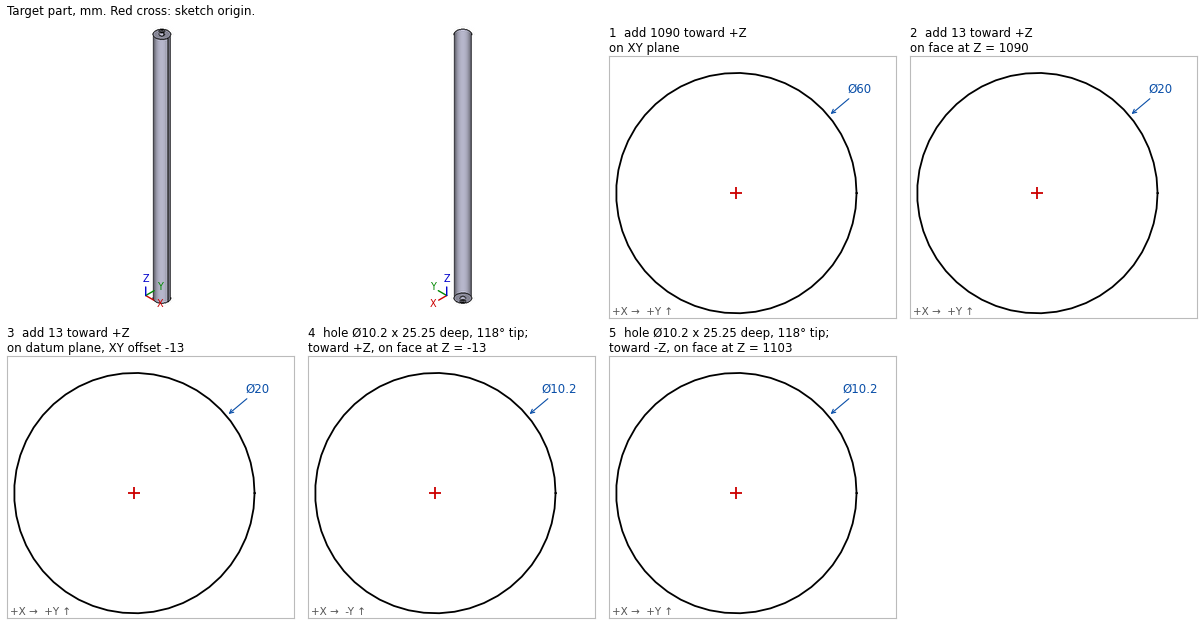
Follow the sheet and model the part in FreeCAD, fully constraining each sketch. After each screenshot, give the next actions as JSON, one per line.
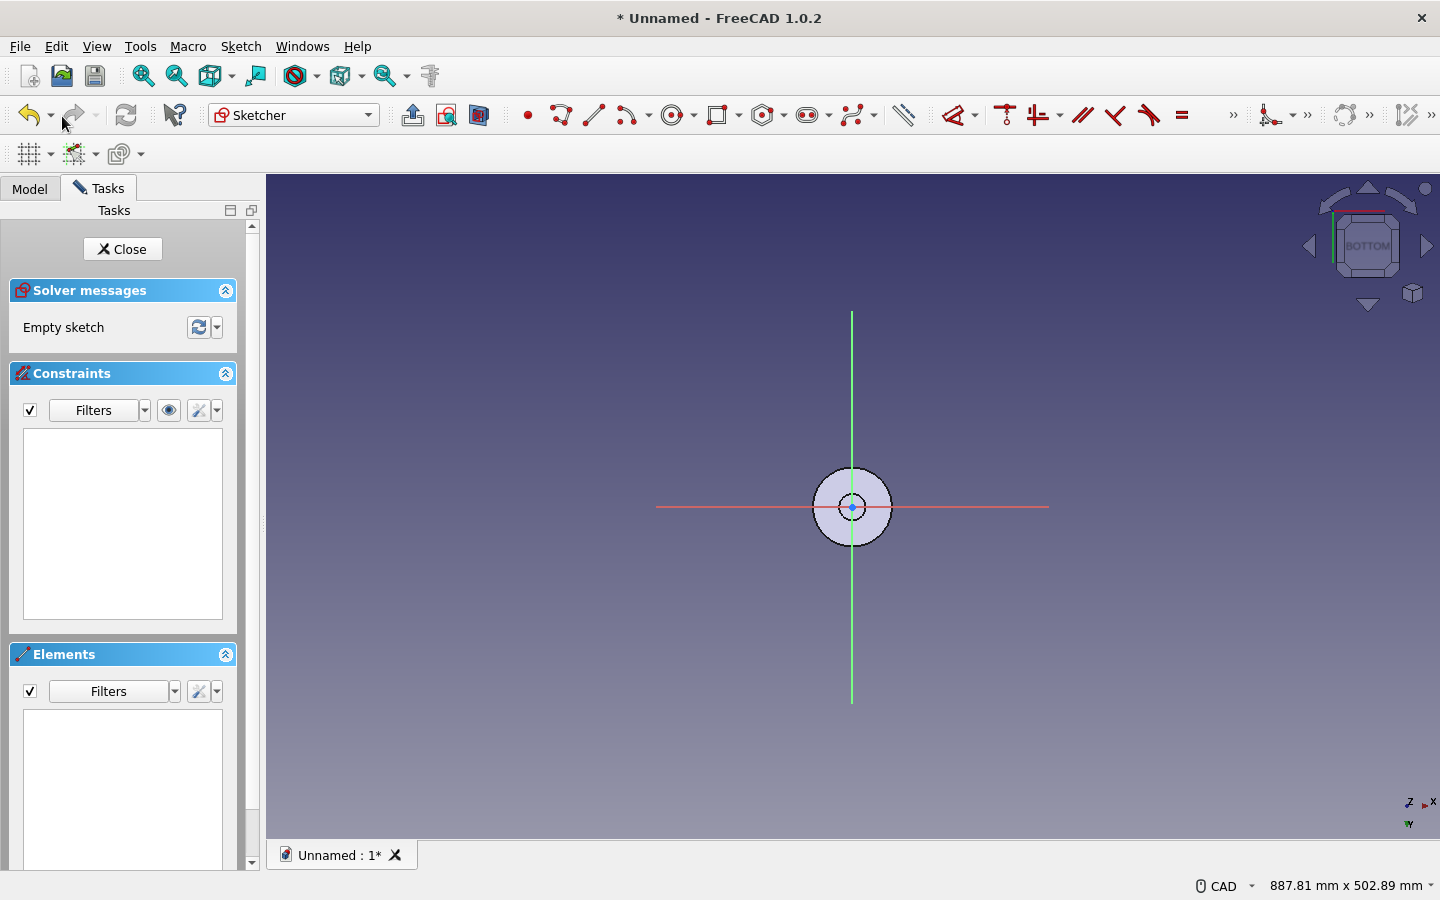
{"action": "scroll", "coordinate": [856, 507], "scroll_direction": "up", "scroll_amount": 15}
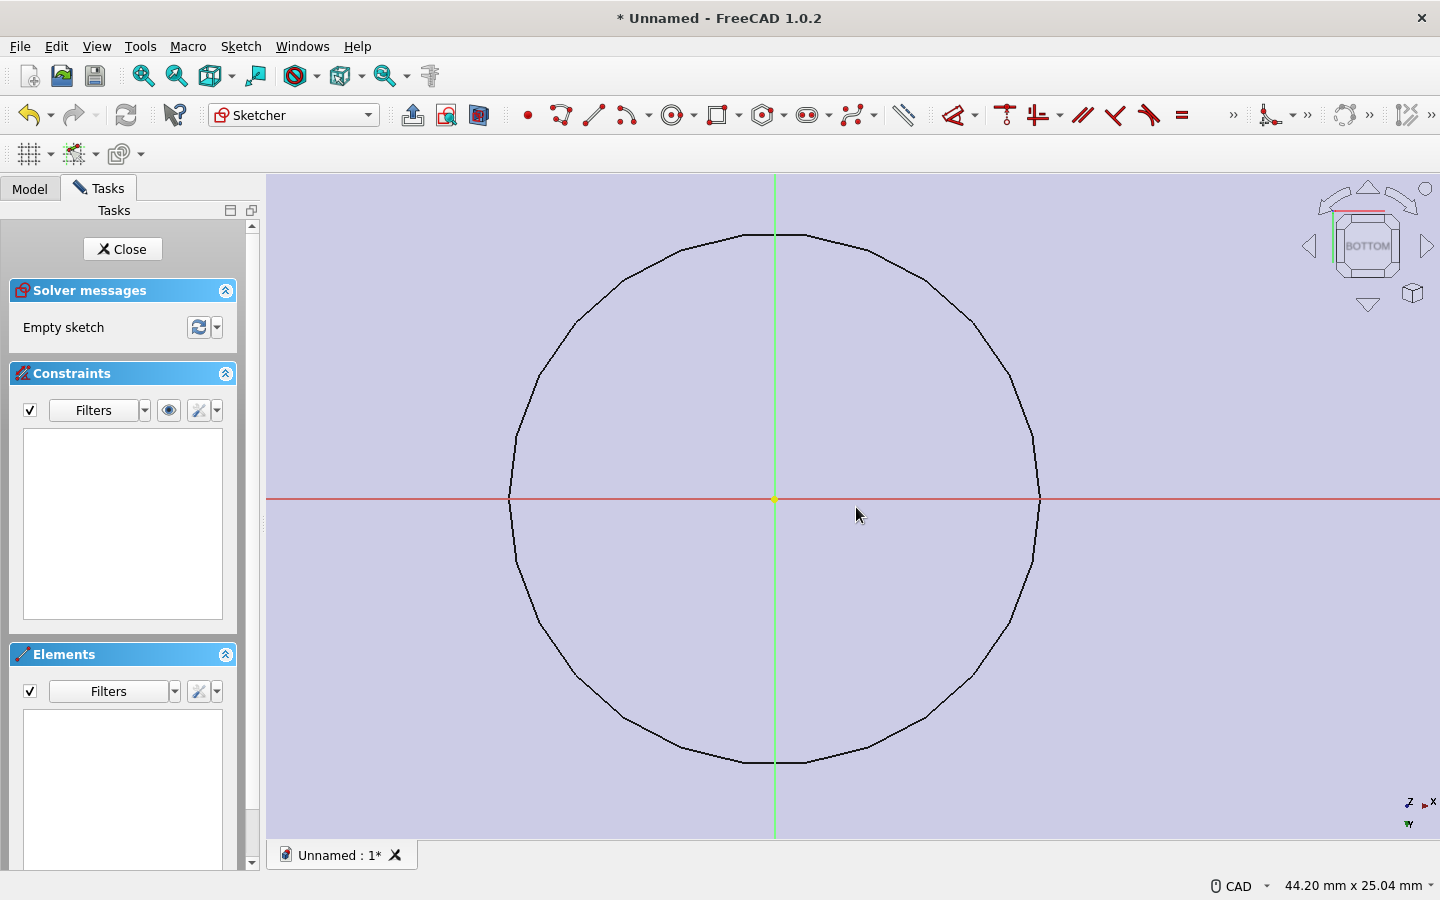
{"action": "scroll", "coordinate": [754, 484], "scroll_direction": "up", "scroll_amount": 2}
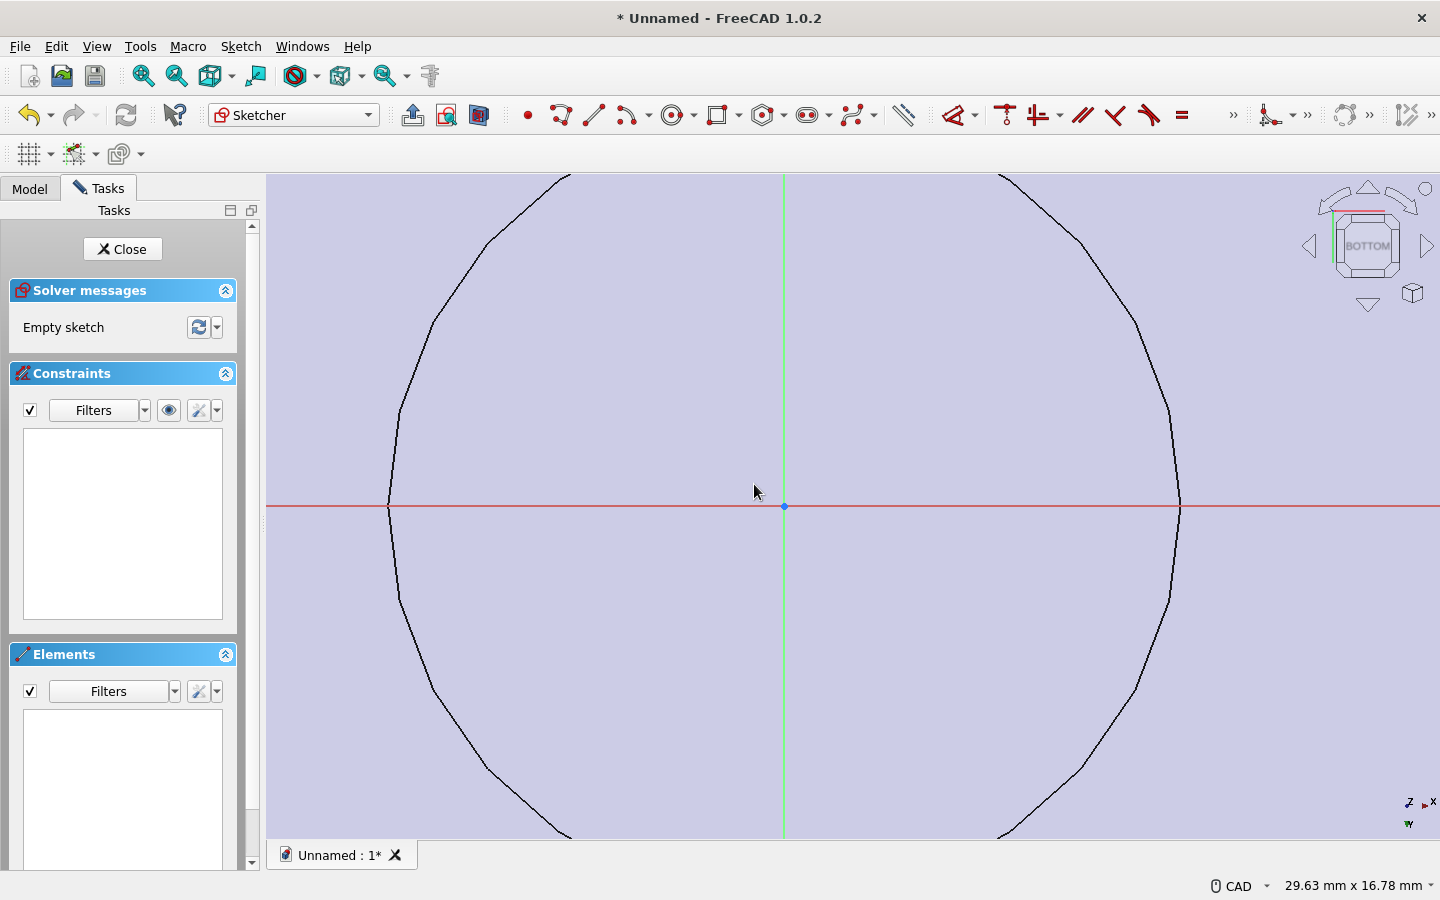
{"action": "key", "text": "g c"}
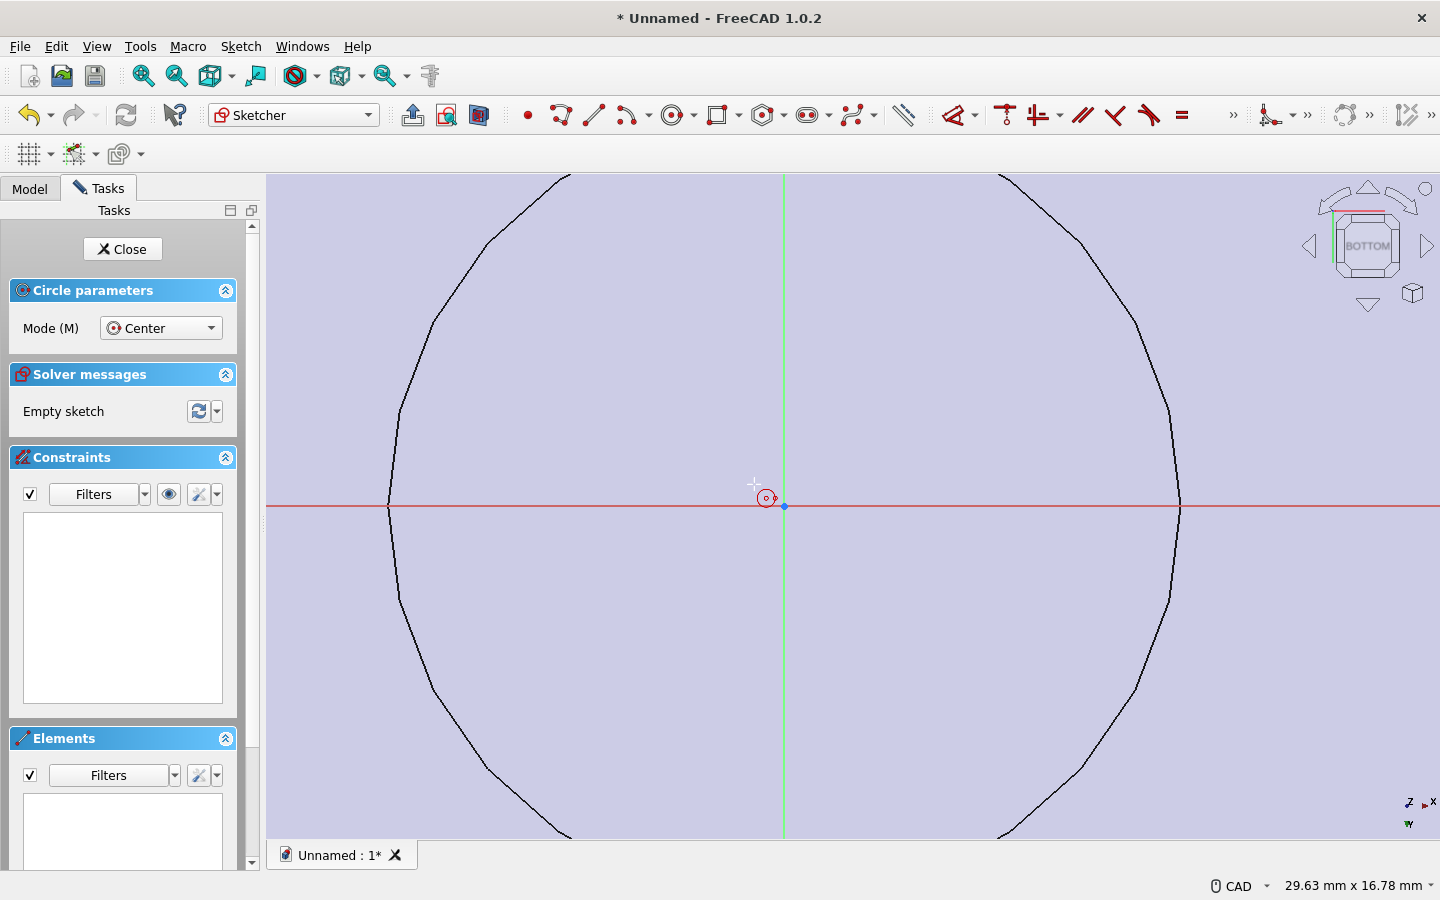
{"action": "left_click", "coordinate": [784, 506]}
{"action": "mouse_move", "coordinate": [927, 363]}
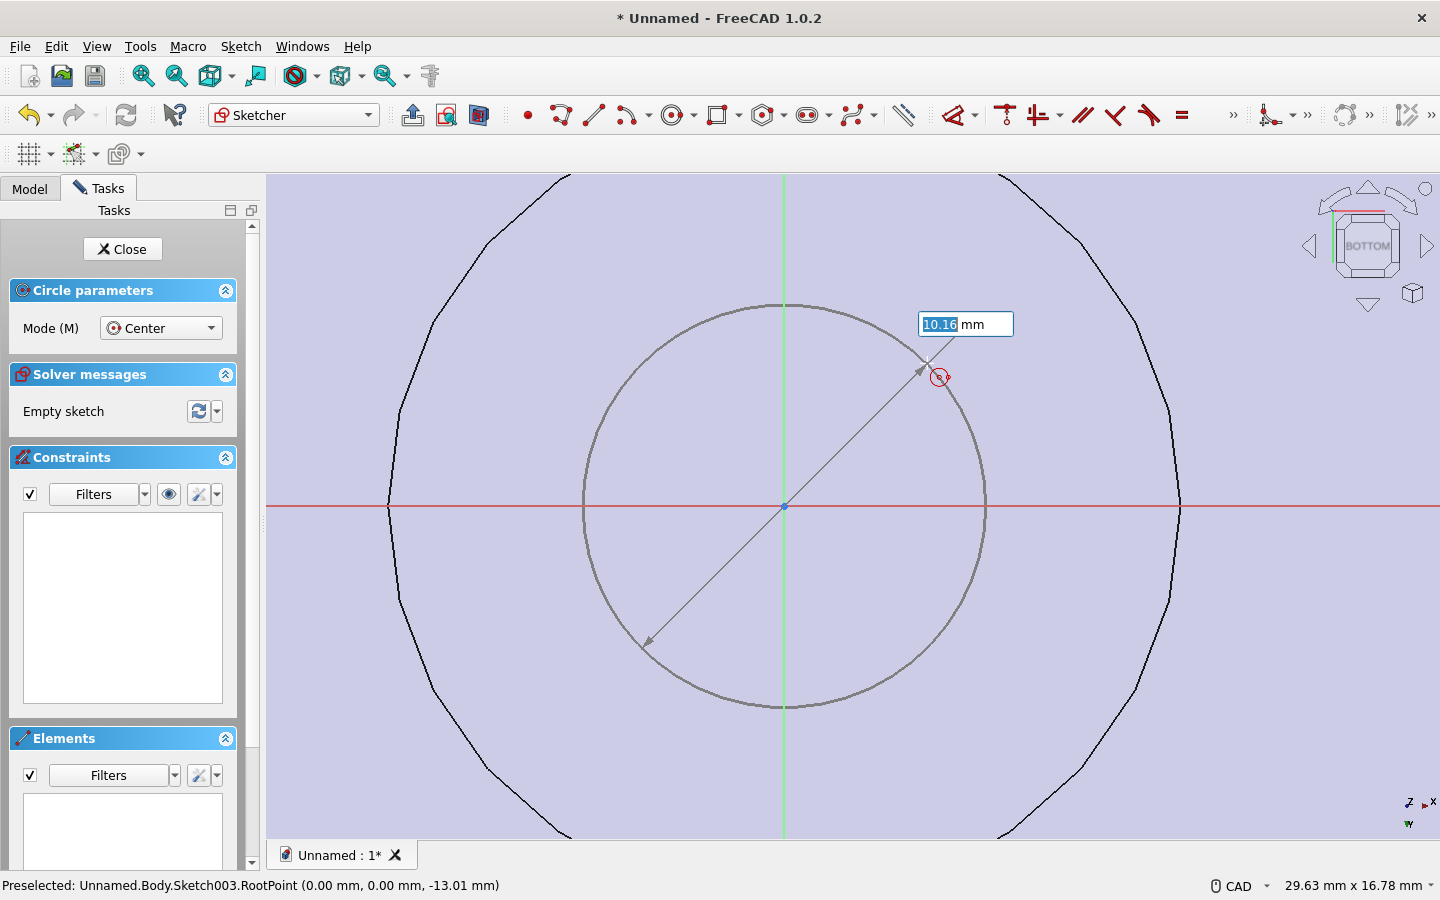
{"action": "type", "text": "10.2"}
{"action": "key", "text": "Return"}
{"action": "key", "text": "Escape"}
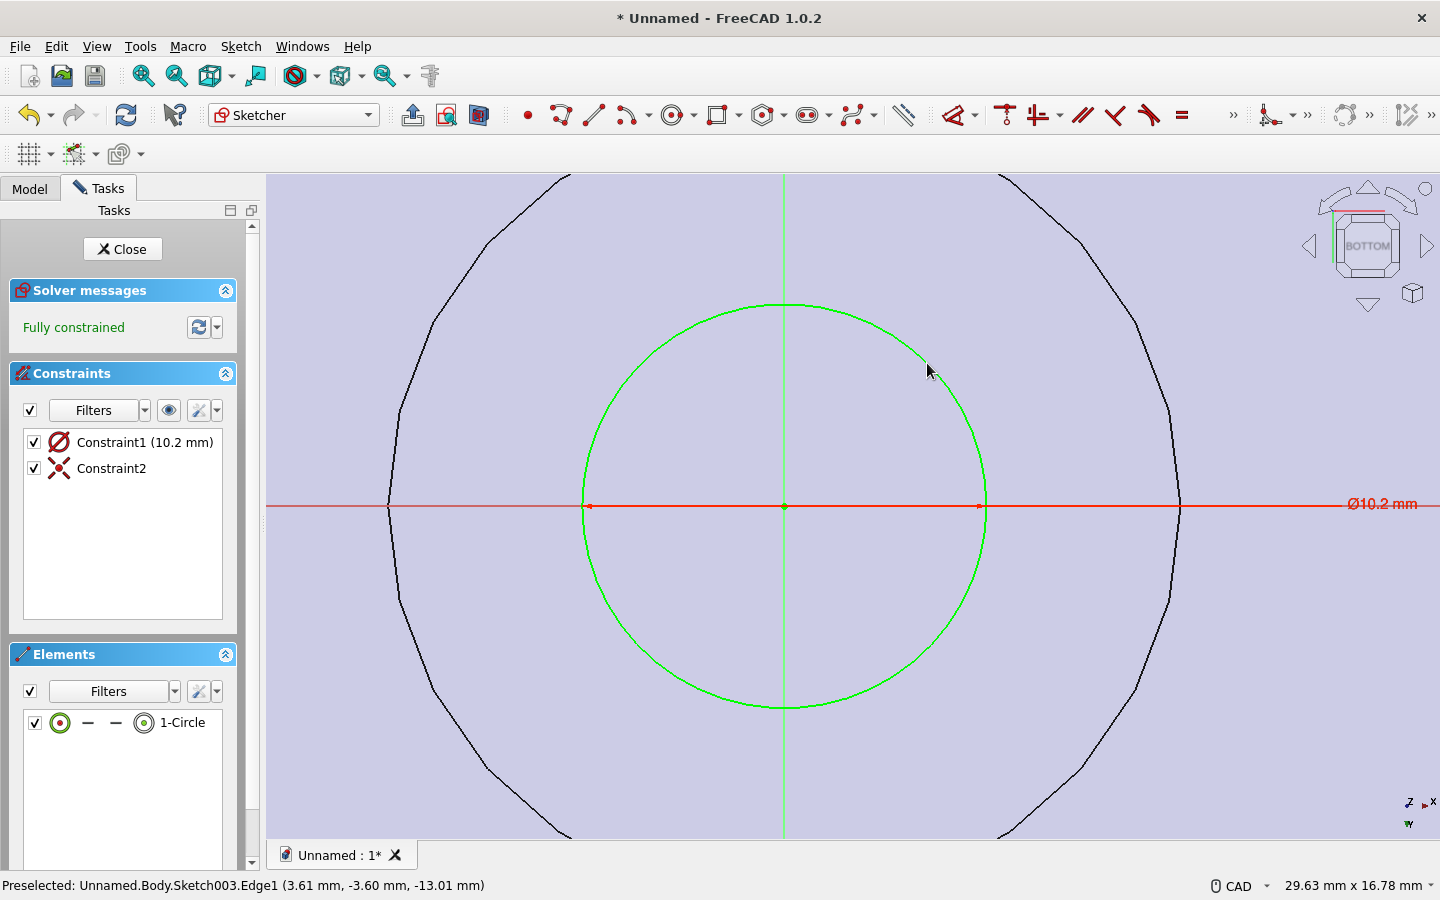
{"action": "left_click", "coordinate": [123, 249]}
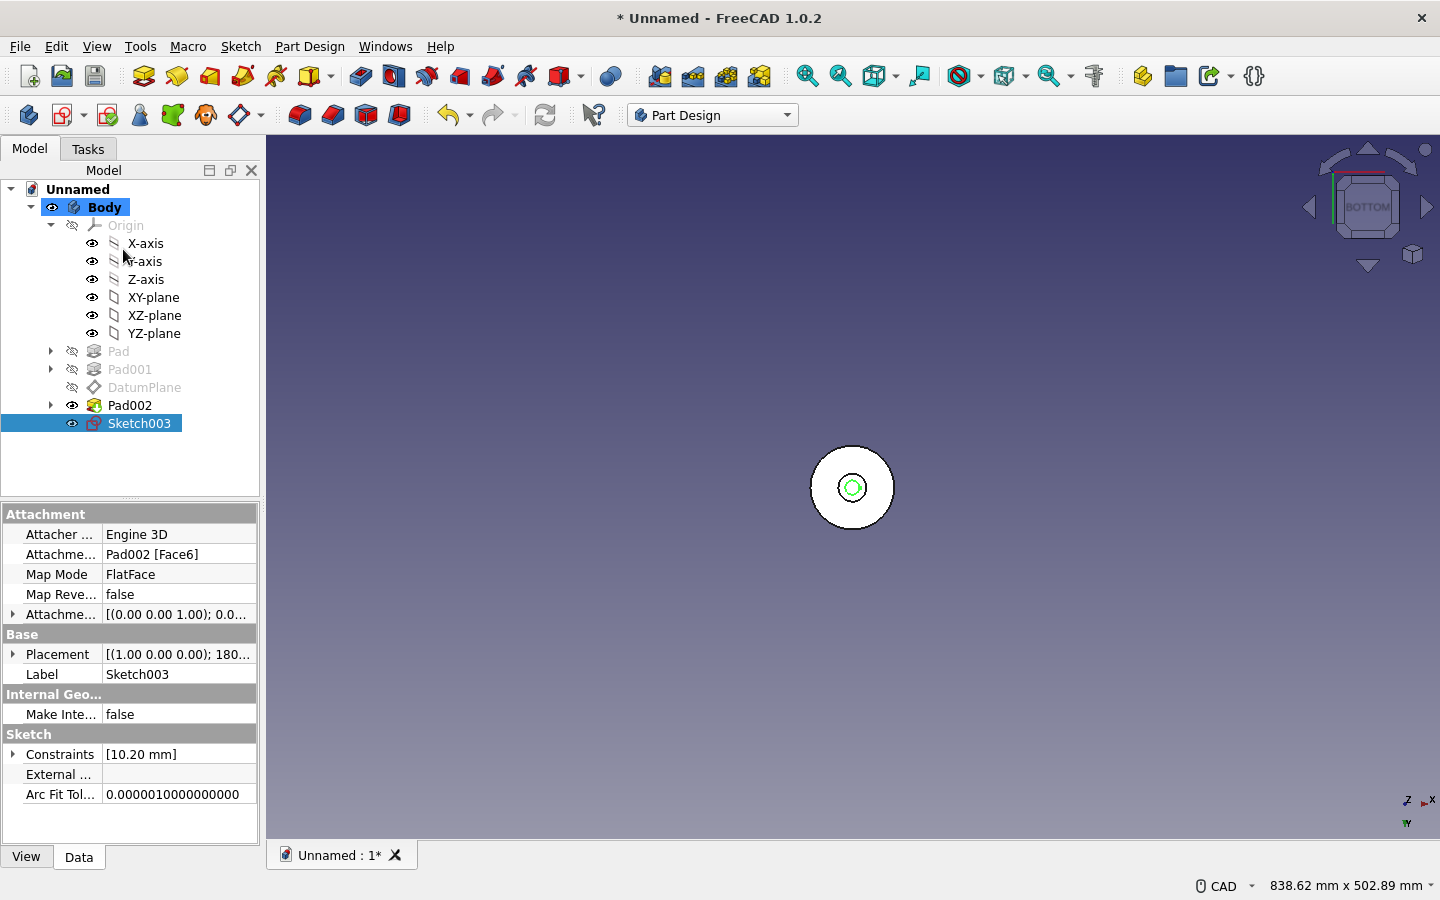
{"action": "left_click", "coordinate": [394, 76]}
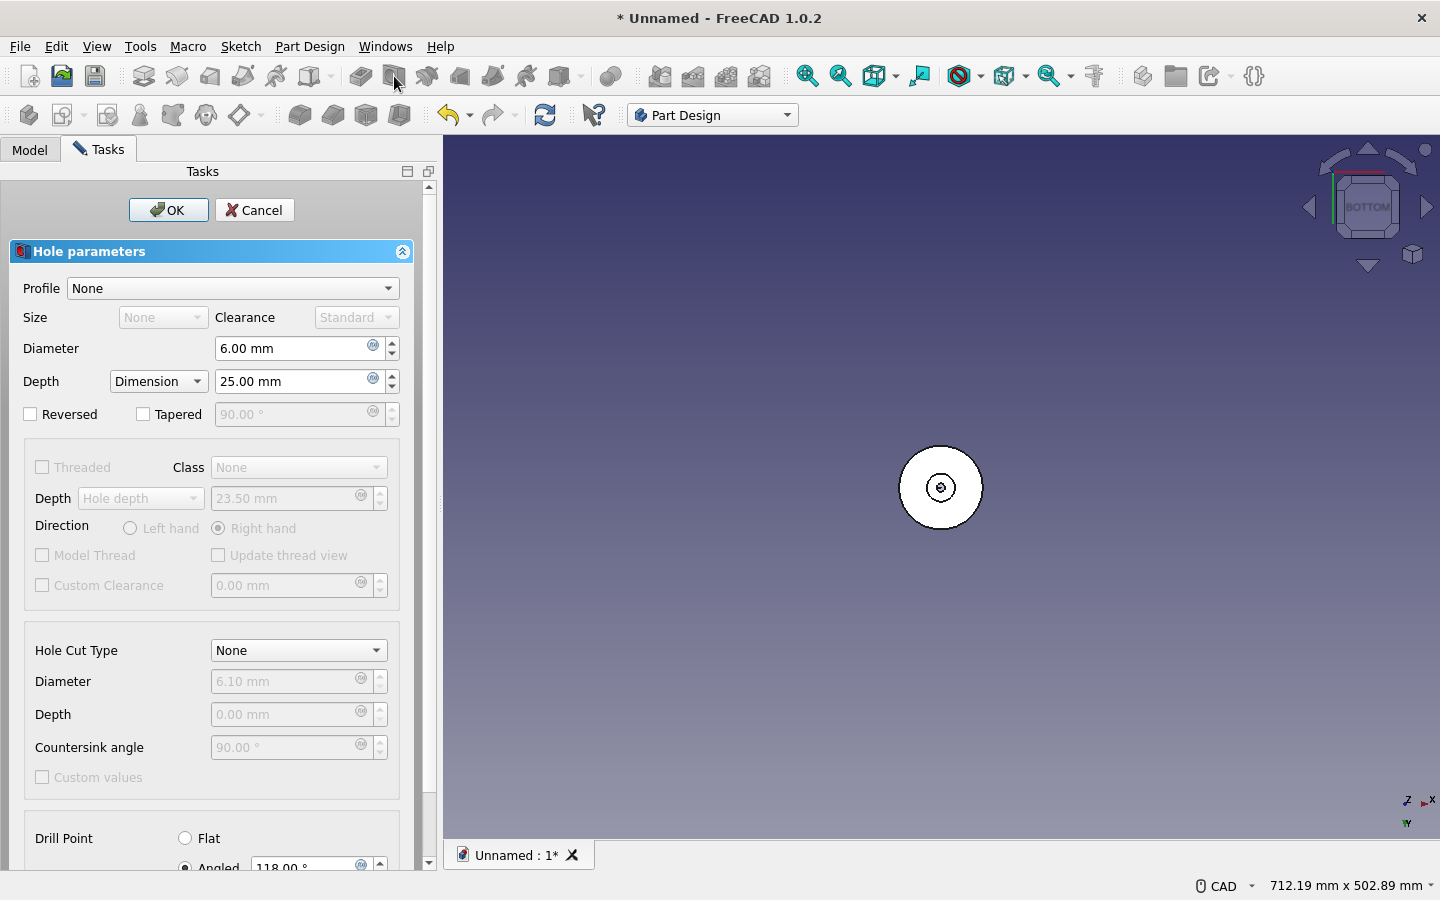
{"action": "triple_click", "coordinate": [300, 348]}